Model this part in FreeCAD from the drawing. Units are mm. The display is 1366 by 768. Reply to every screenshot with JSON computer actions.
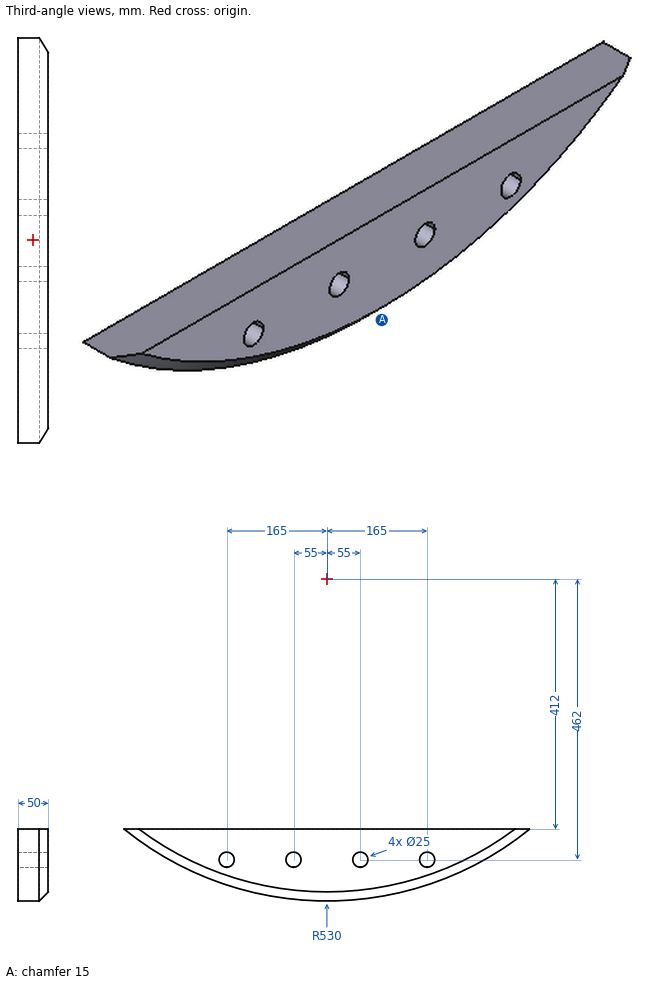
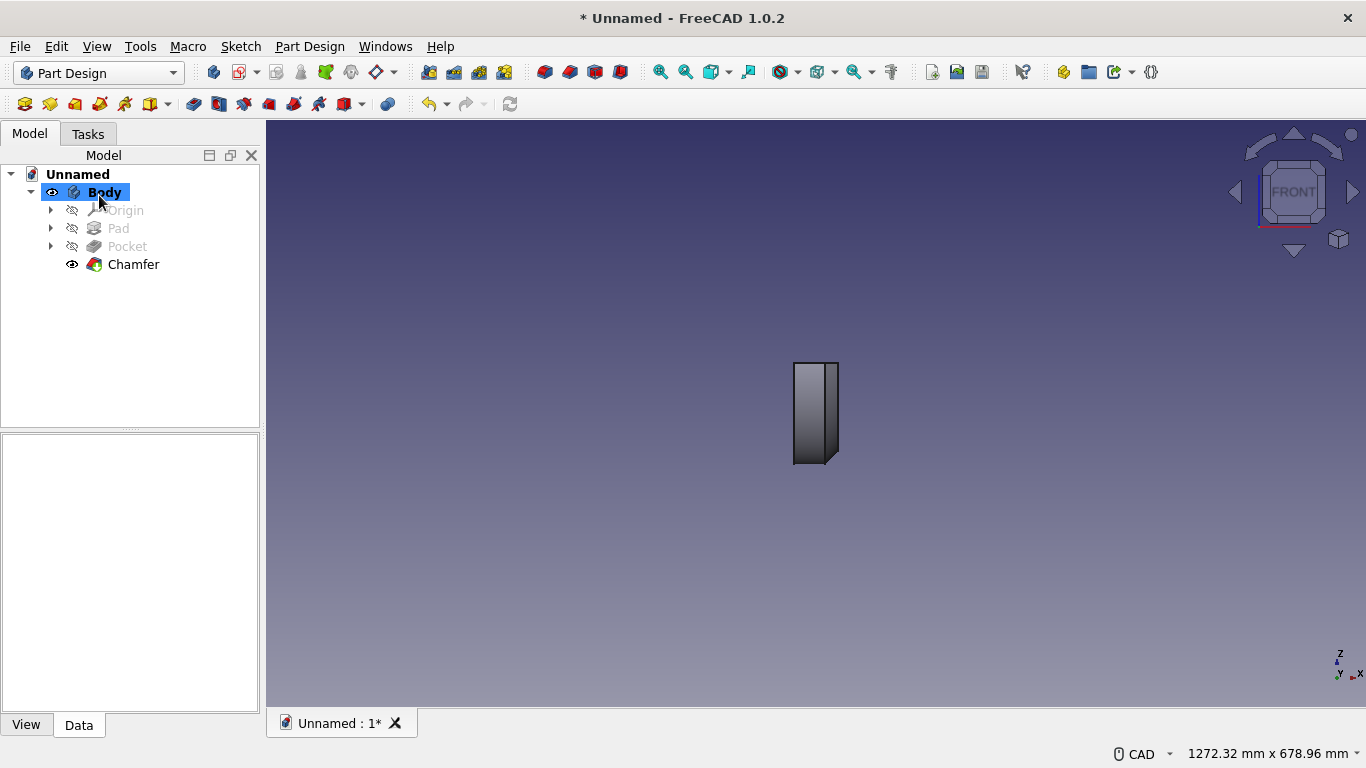
{"action": "key", "text": "0"}